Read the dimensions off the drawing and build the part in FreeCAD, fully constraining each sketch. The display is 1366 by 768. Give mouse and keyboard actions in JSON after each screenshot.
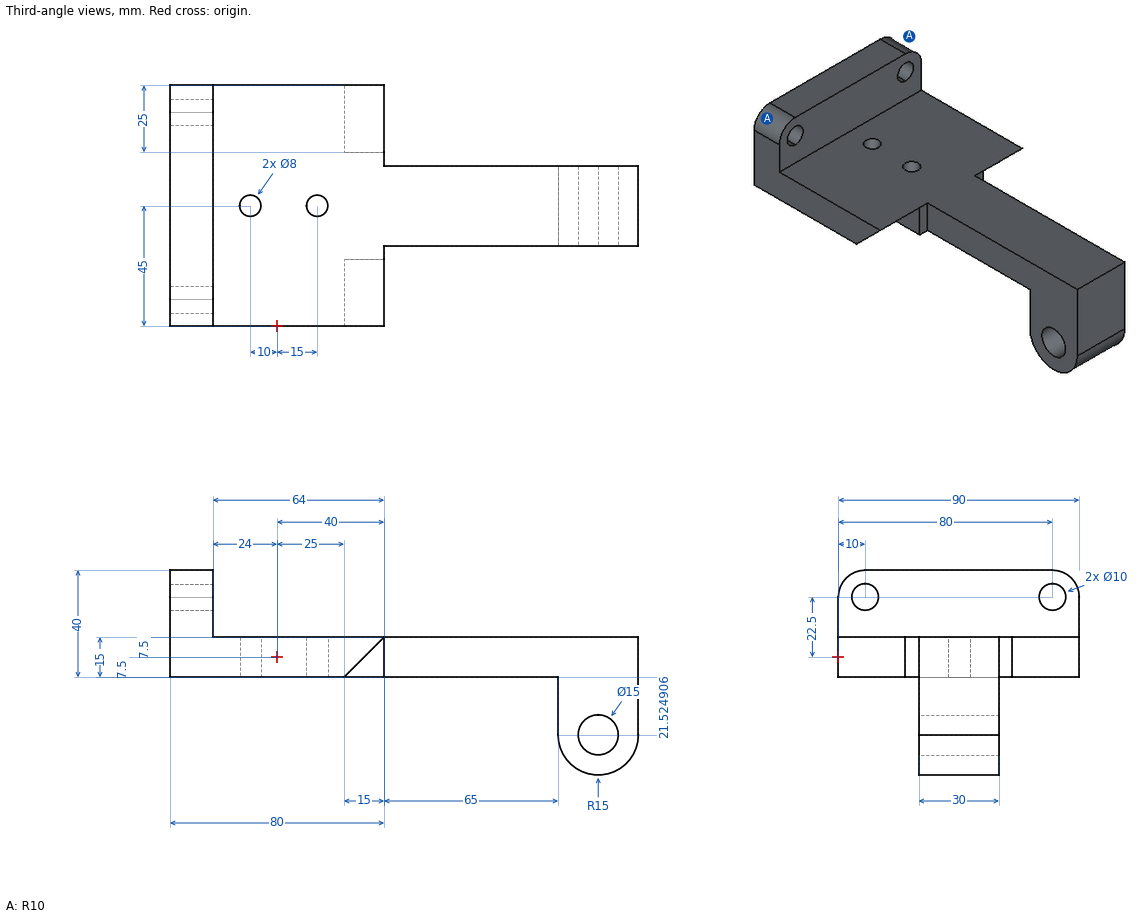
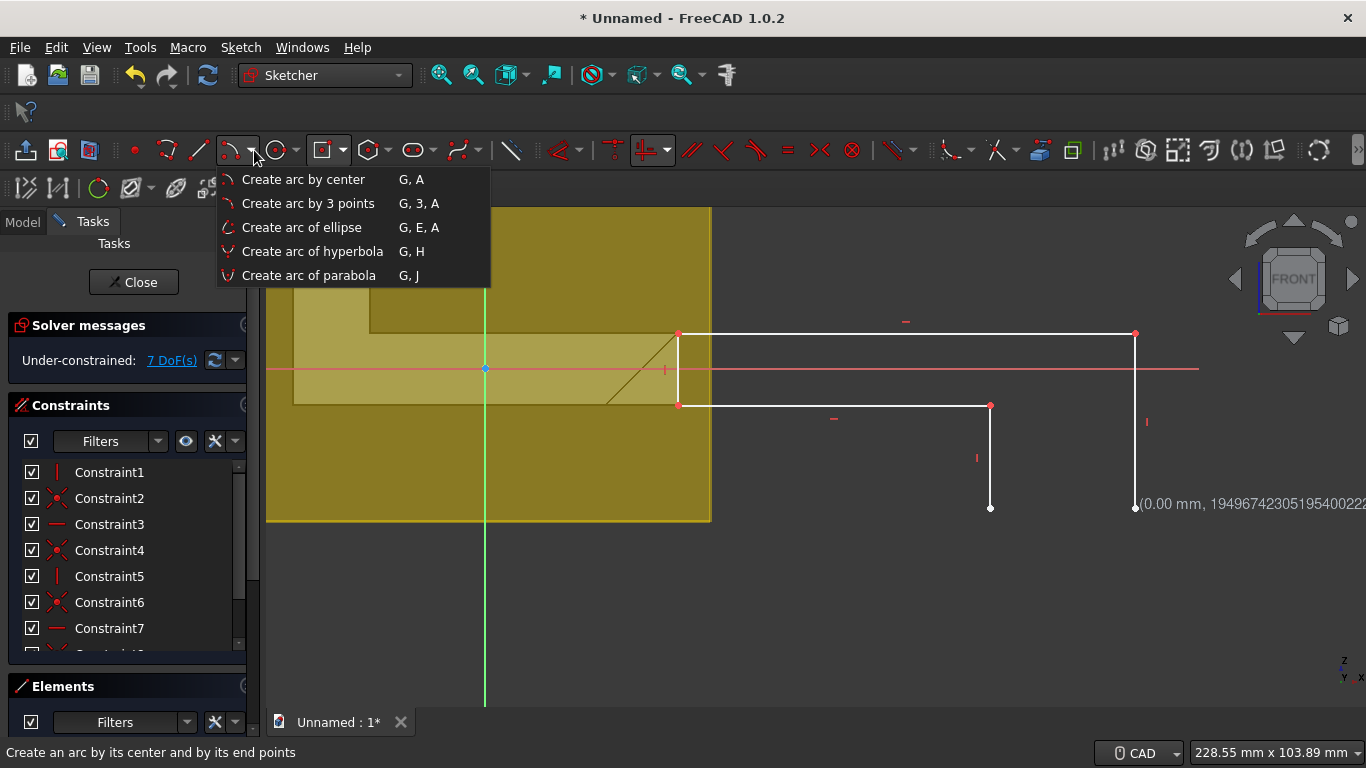
{"action": "left_click", "coordinate": [354, 203]}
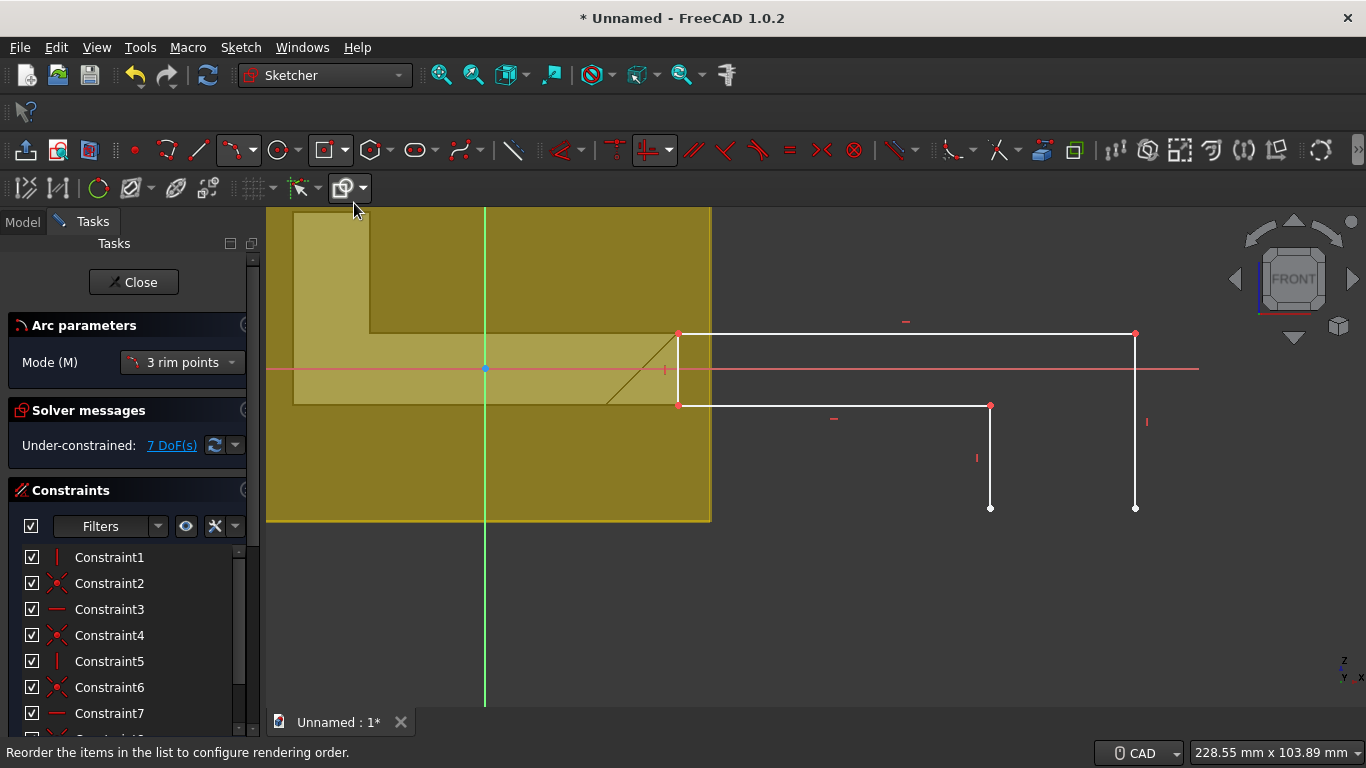
{"action": "left_click", "coordinate": [1135, 509]}
{"action": "left_click", "coordinate": [990, 509]}
{"action": "left_click", "coordinate": [1063, 581]}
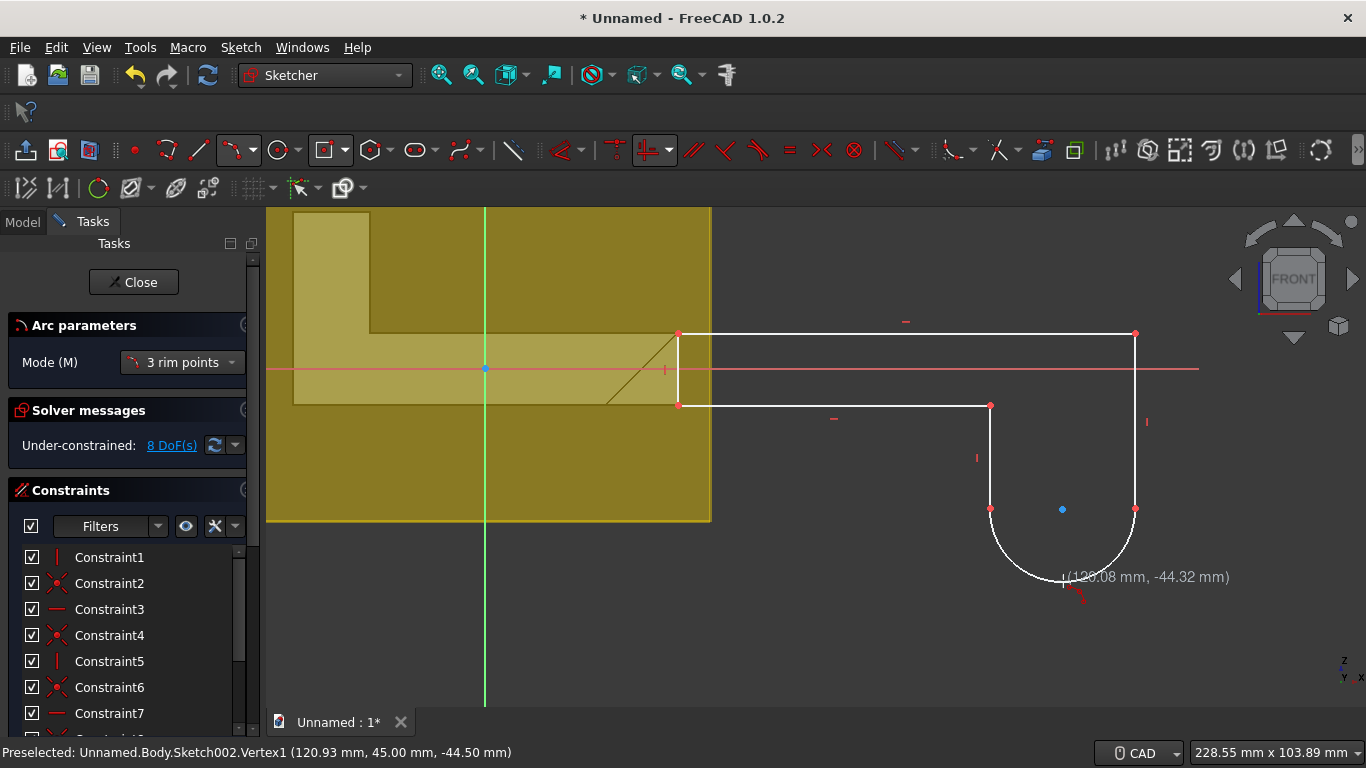
{"action": "left_click", "coordinate": [278, 150]}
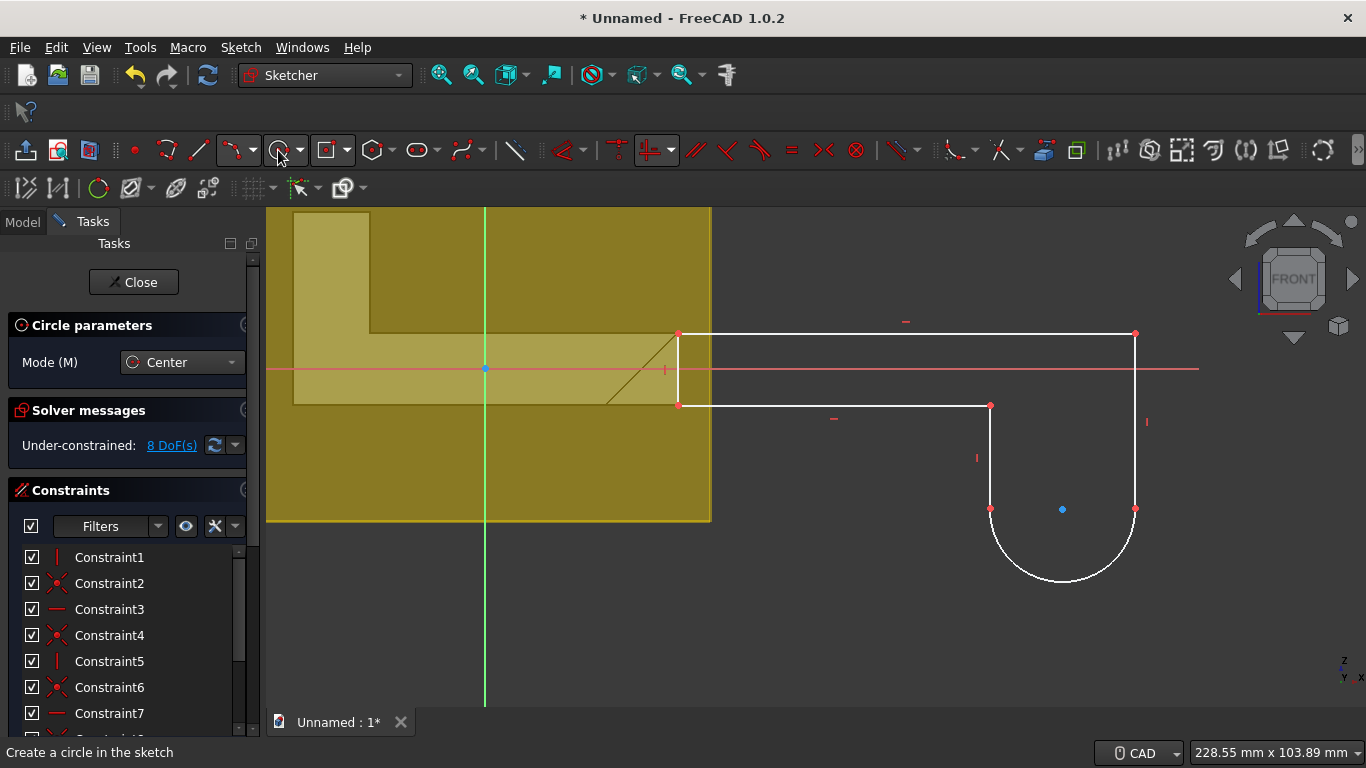
{"action": "left_click", "coordinate": [1063, 508]}
{"action": "left_click", "coordinate": [1088, 483]}
{"action": "key", "text": "Escape"}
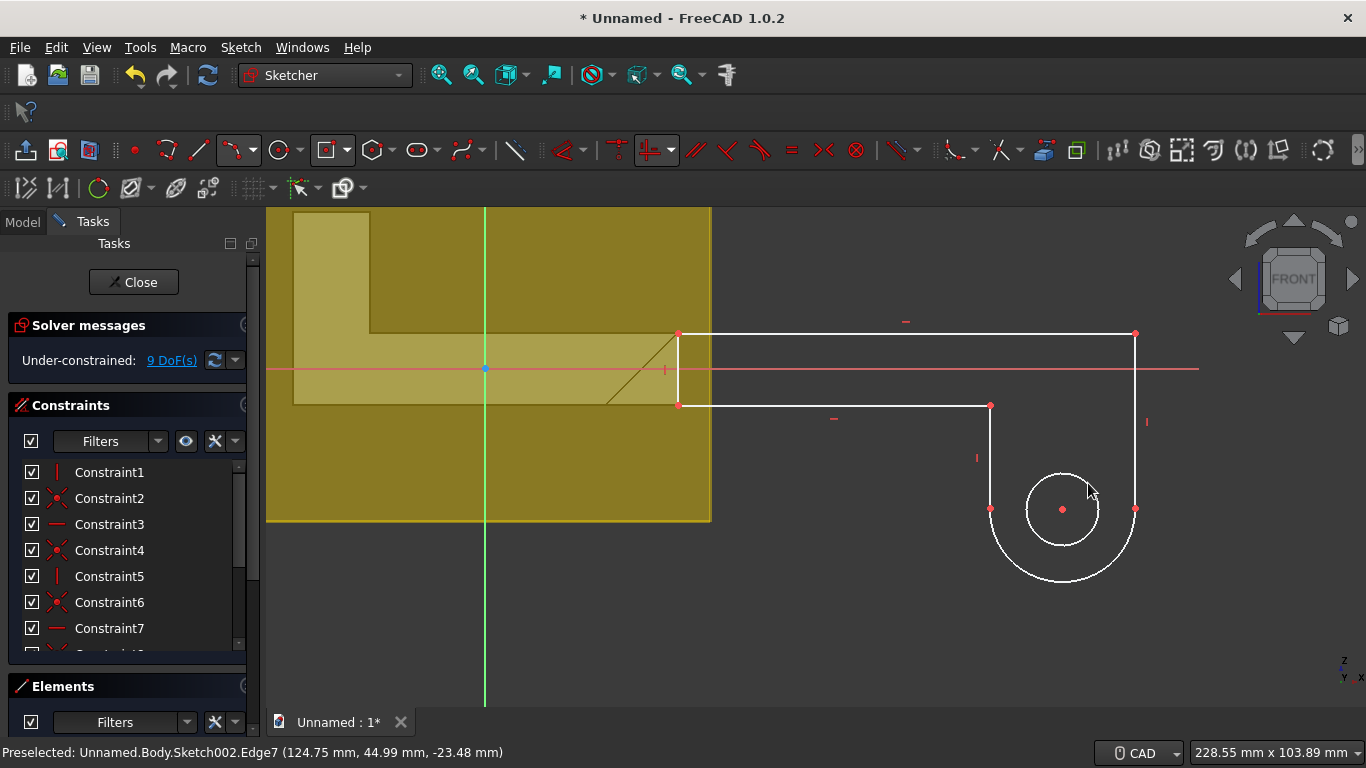
{"action": "left_click", "coordinate": [990, 478]}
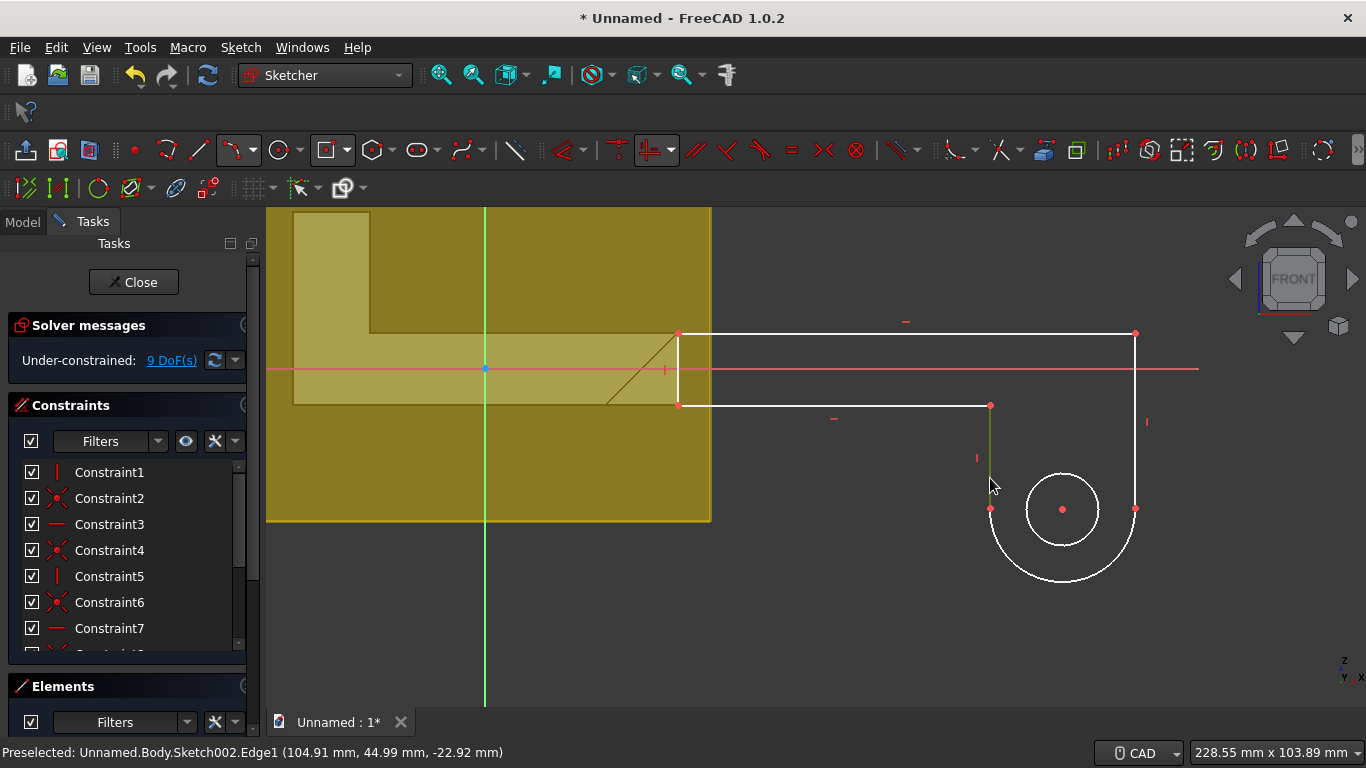
{"action": "left_click", "coordinate": [1020, 568]}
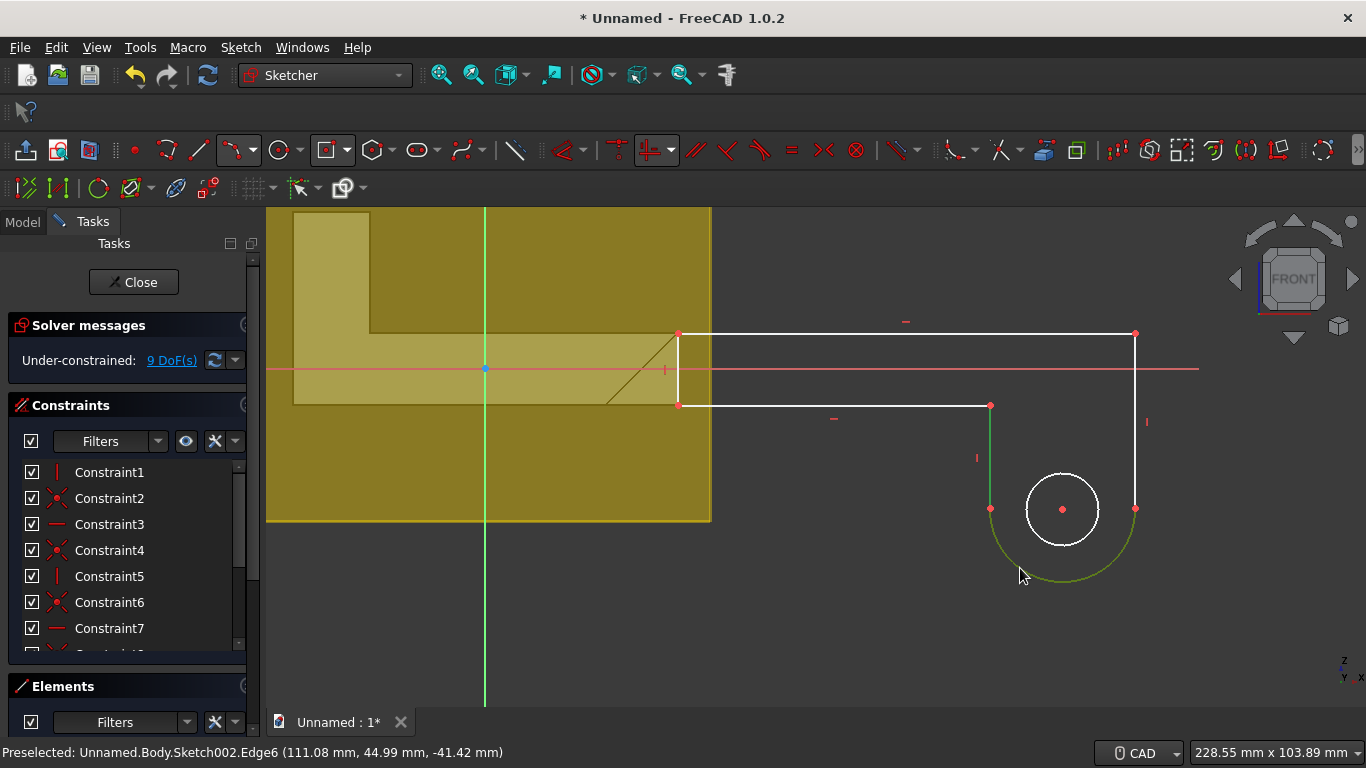
{"action": "left_click", "coordinate": [760, 150]}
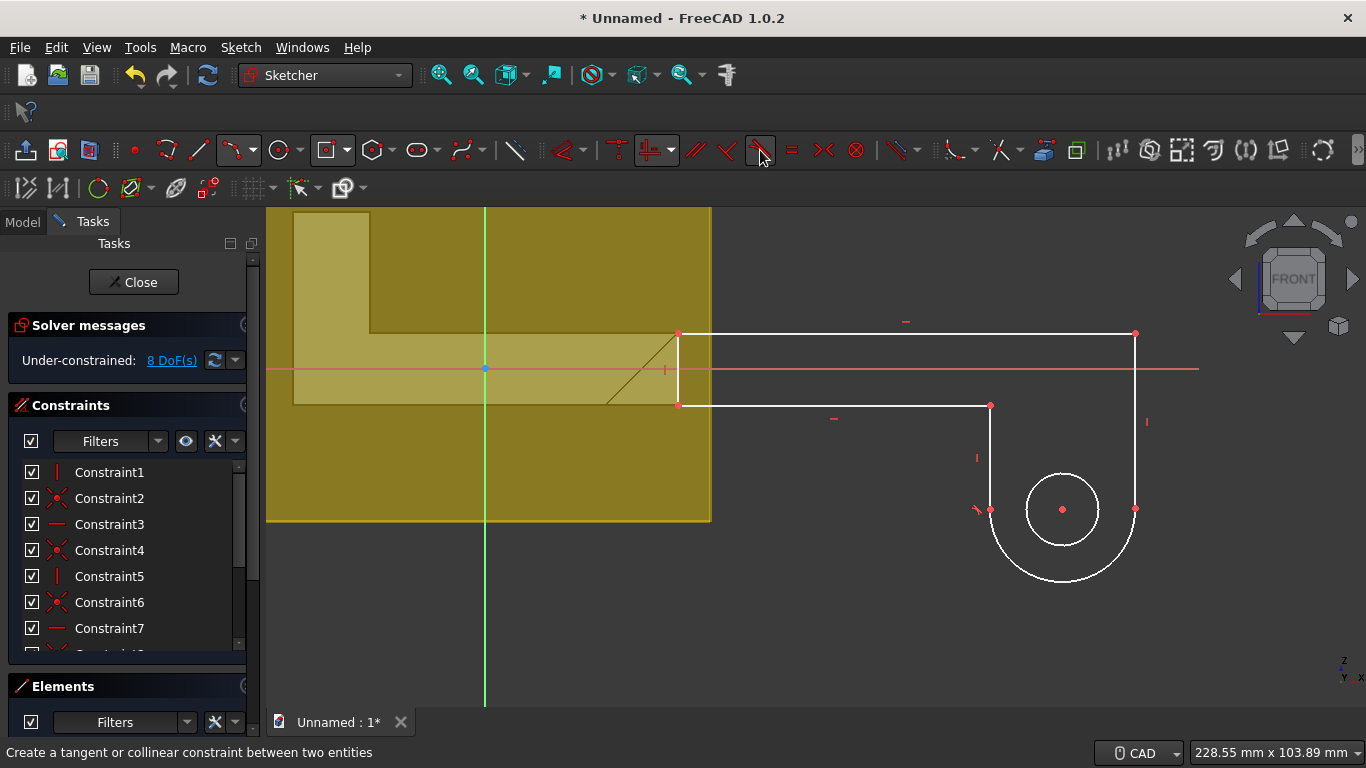
{"action": "left_click", "coordinate": [1135, 387]}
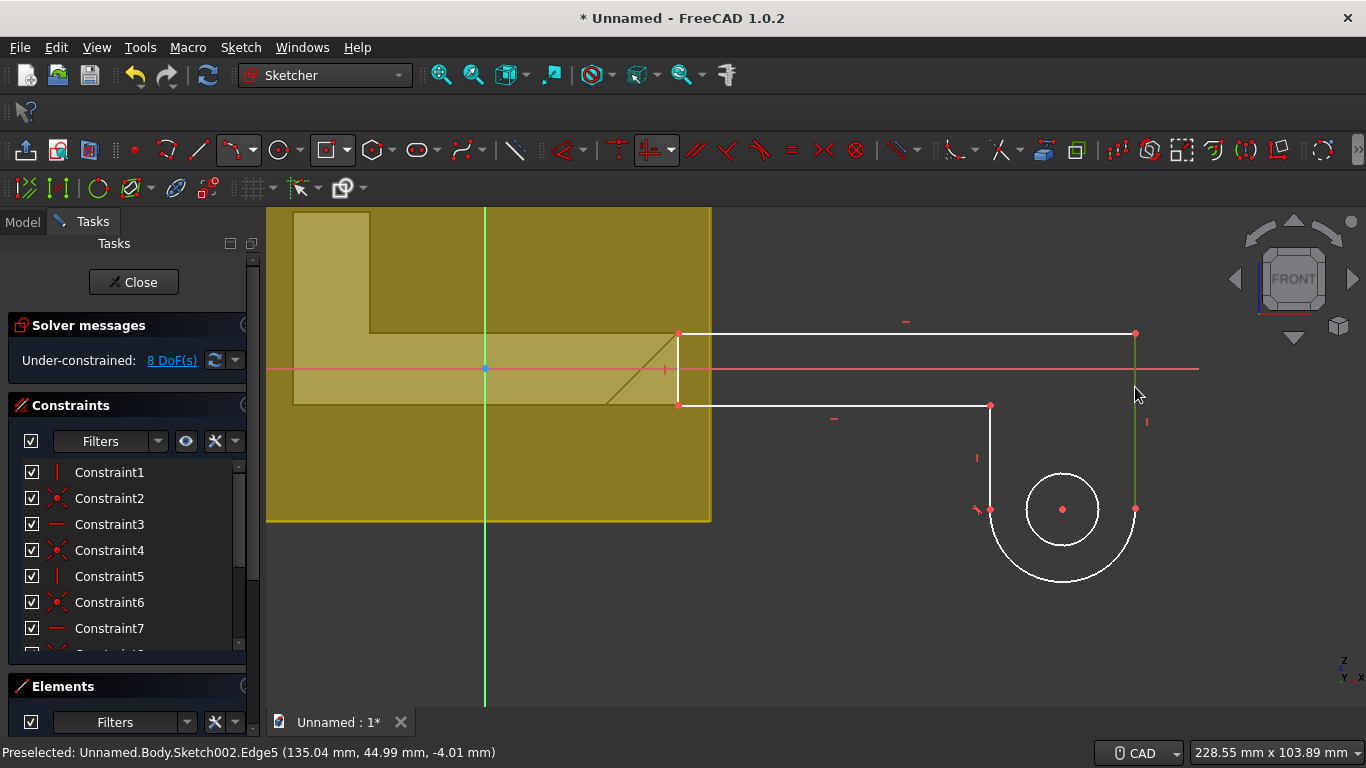
{"action": "left_click", "coordinate": [1020, 568]}